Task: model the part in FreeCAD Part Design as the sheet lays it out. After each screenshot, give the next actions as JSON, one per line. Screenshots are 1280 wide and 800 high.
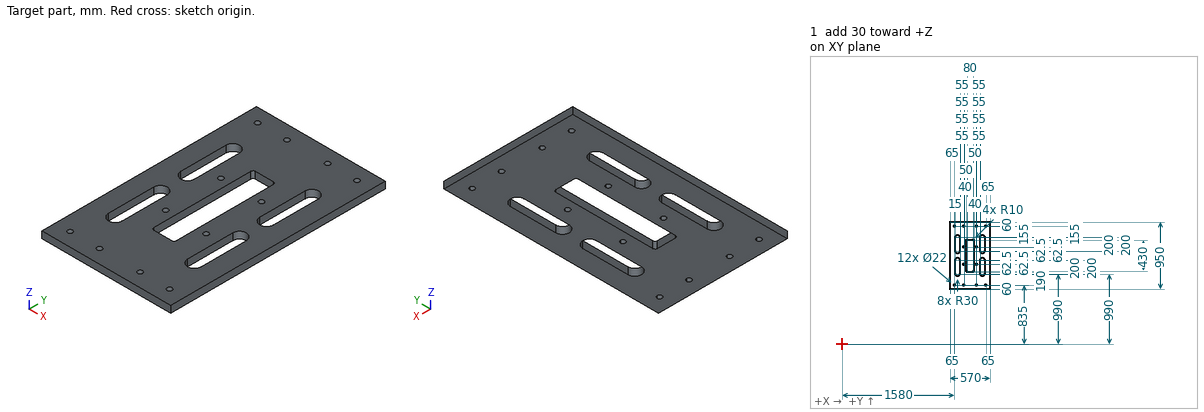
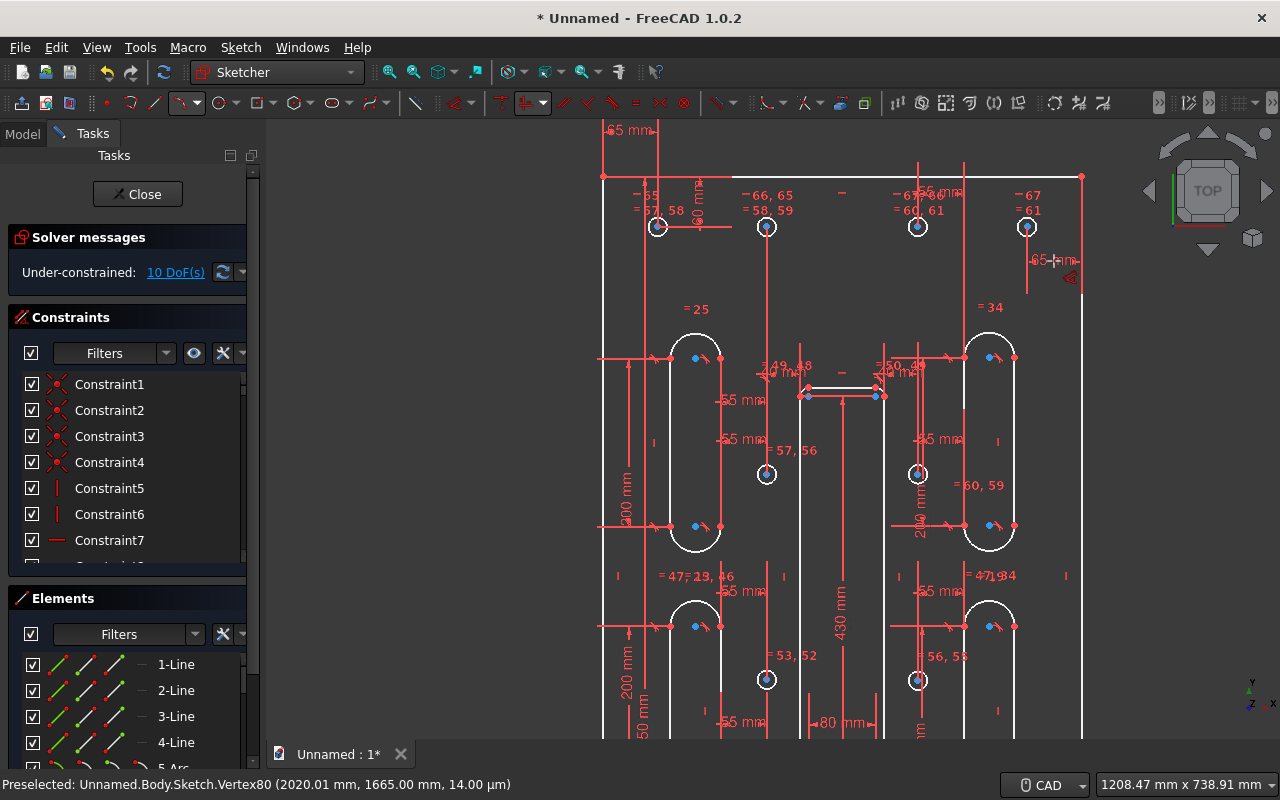
{"action": "scroll", "coordinate": [919, 226], "scroll_direction": "down", "scroll_amount": 6}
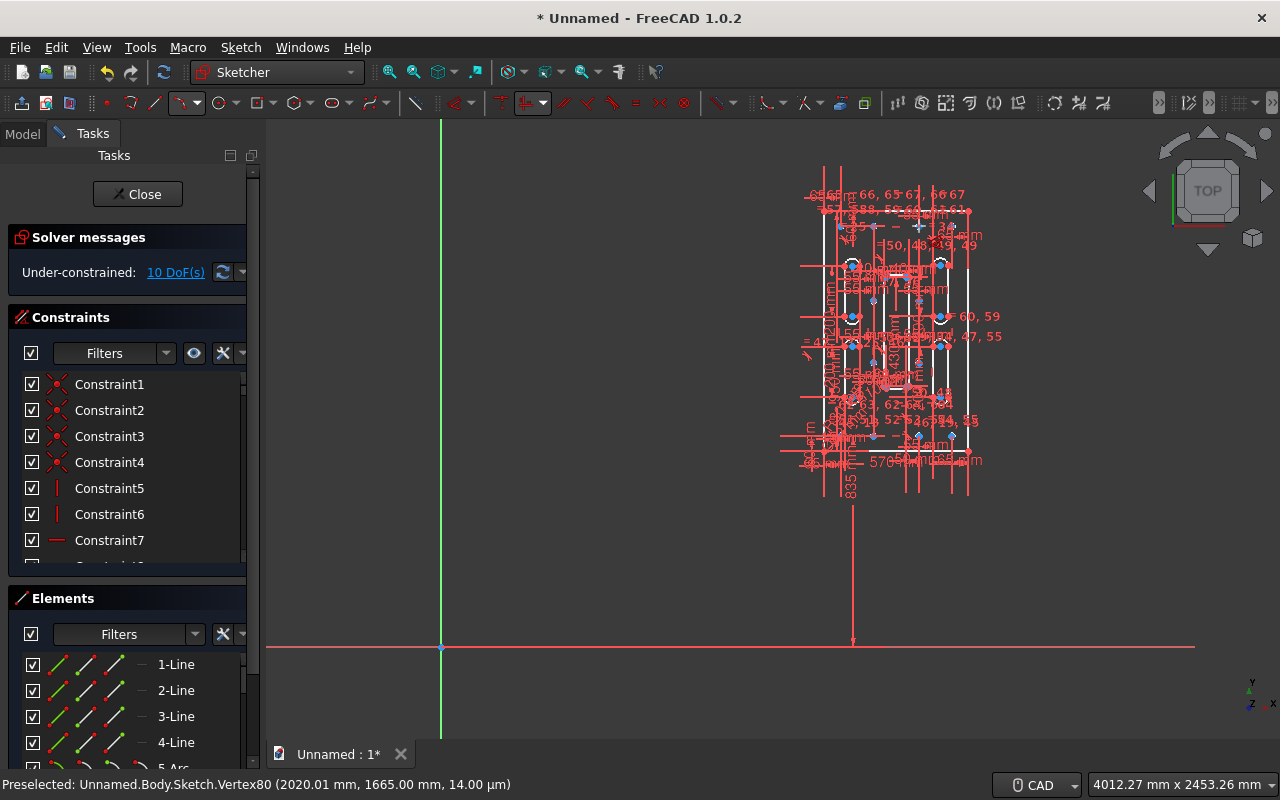
{"action": "scroll", "coordinate": [845, 397], "scroll_direction": "up", "scroll_amount": 3}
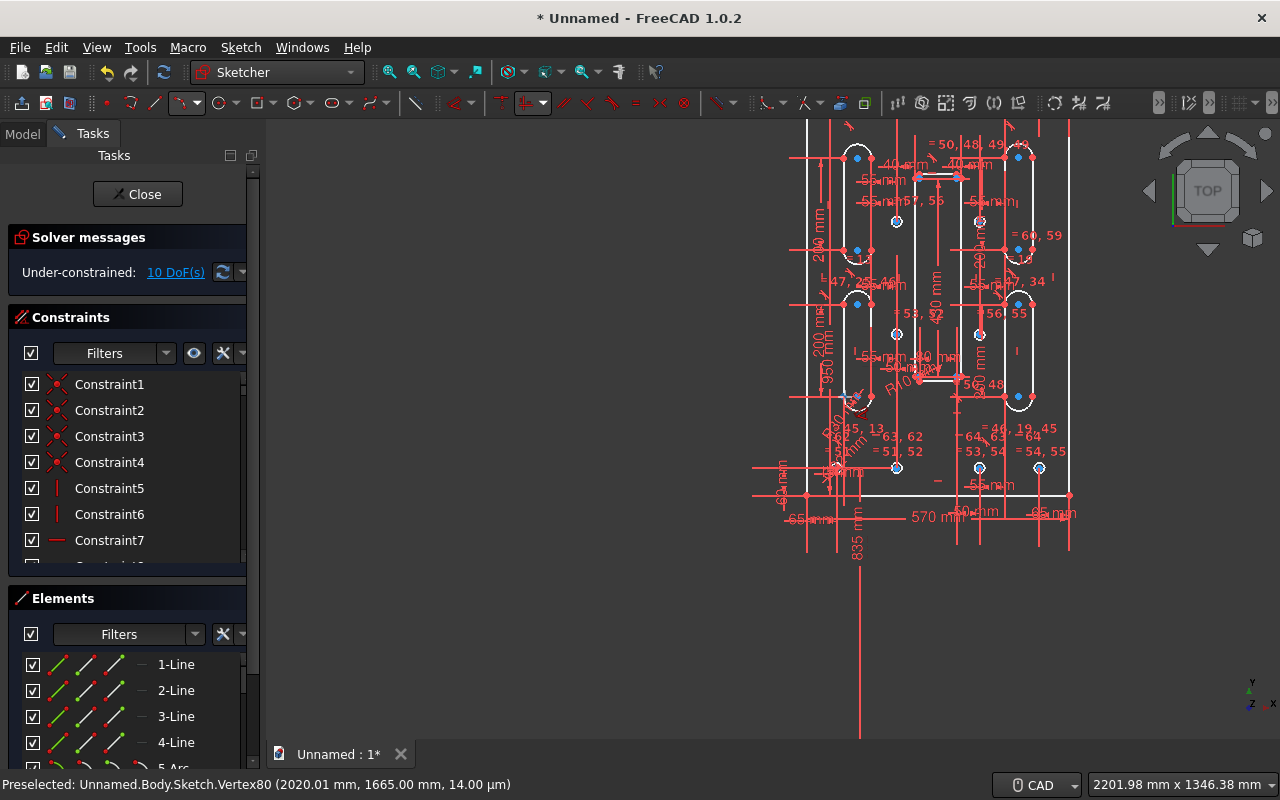
{"action": "left_click", "coordinate": [844, 397]}
{"action": "left_click", "coordinate": [878, 554]}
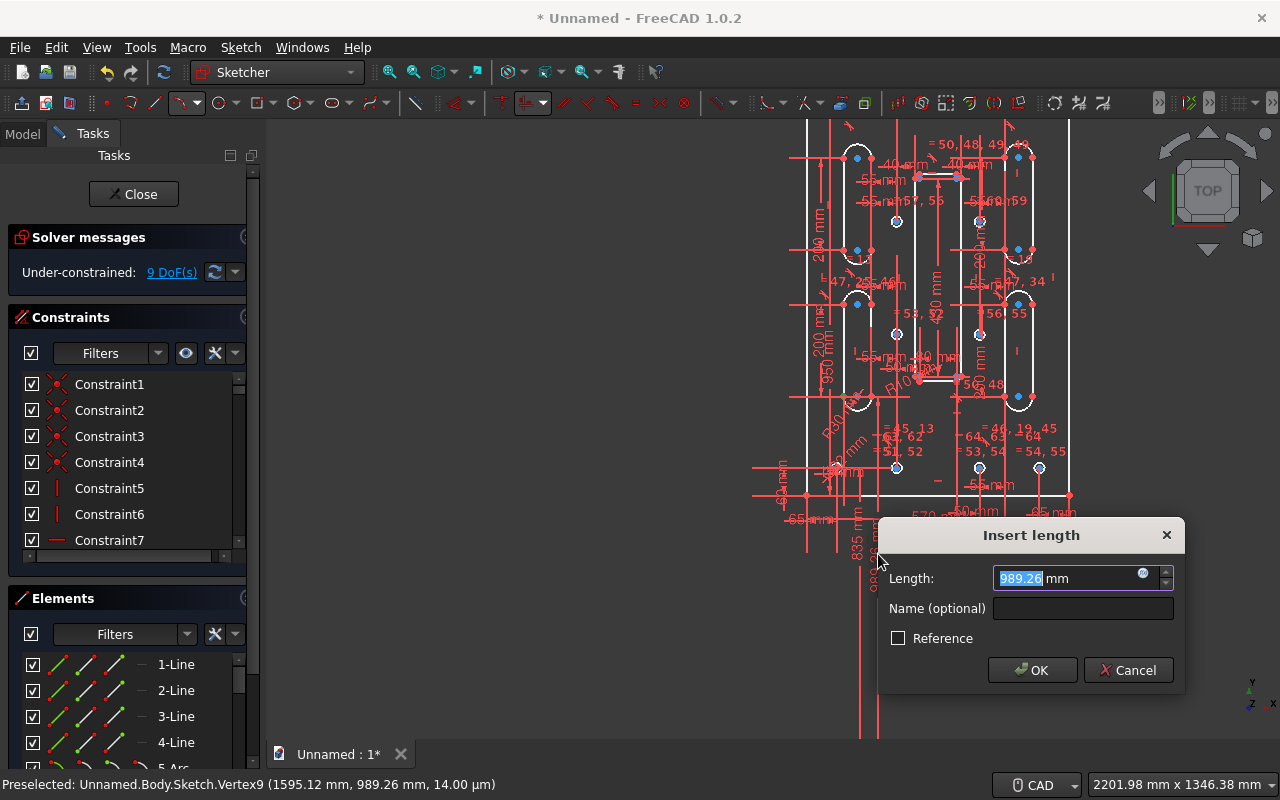
{"action": "type", "text": "990"}
{"action": "key", "text": "Return"}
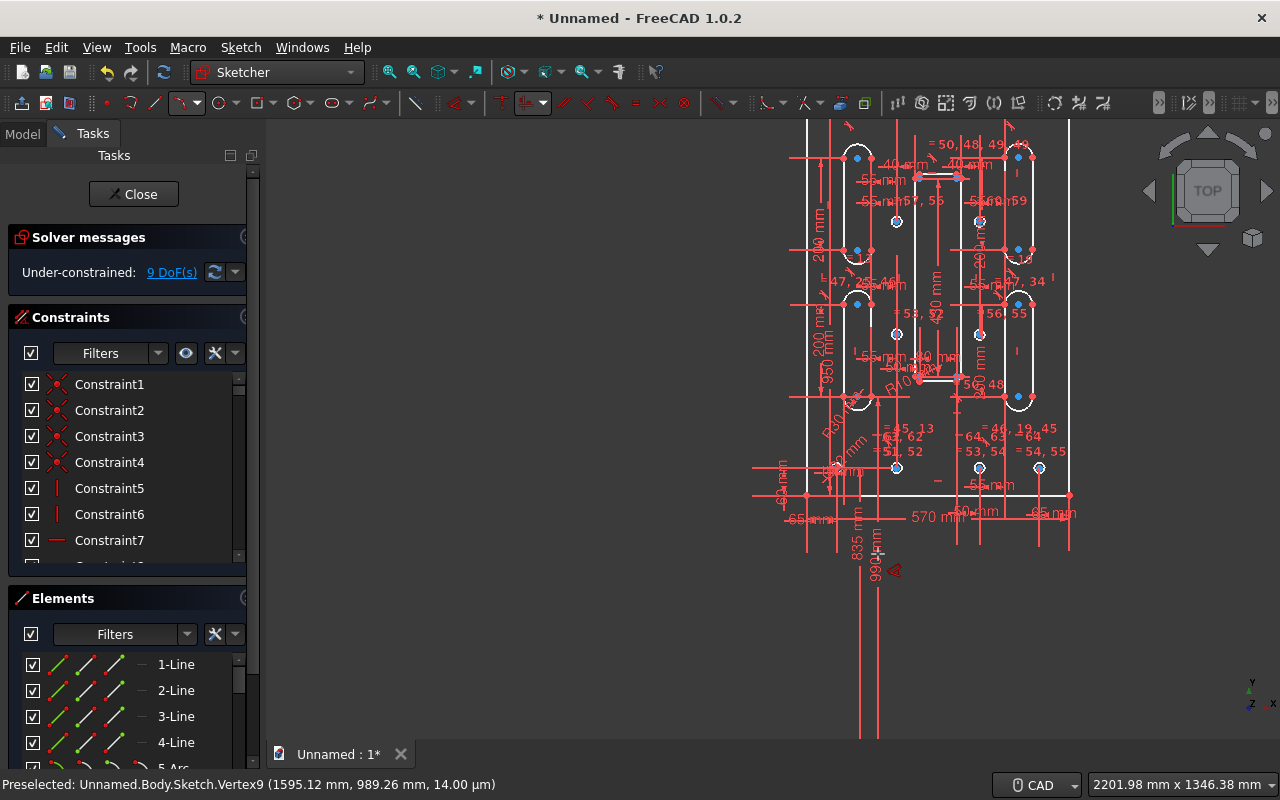
{"action": "left_click", "coordinate": [1005, 397]}
{"action": "left_click", "coordinate": [1039, 554]}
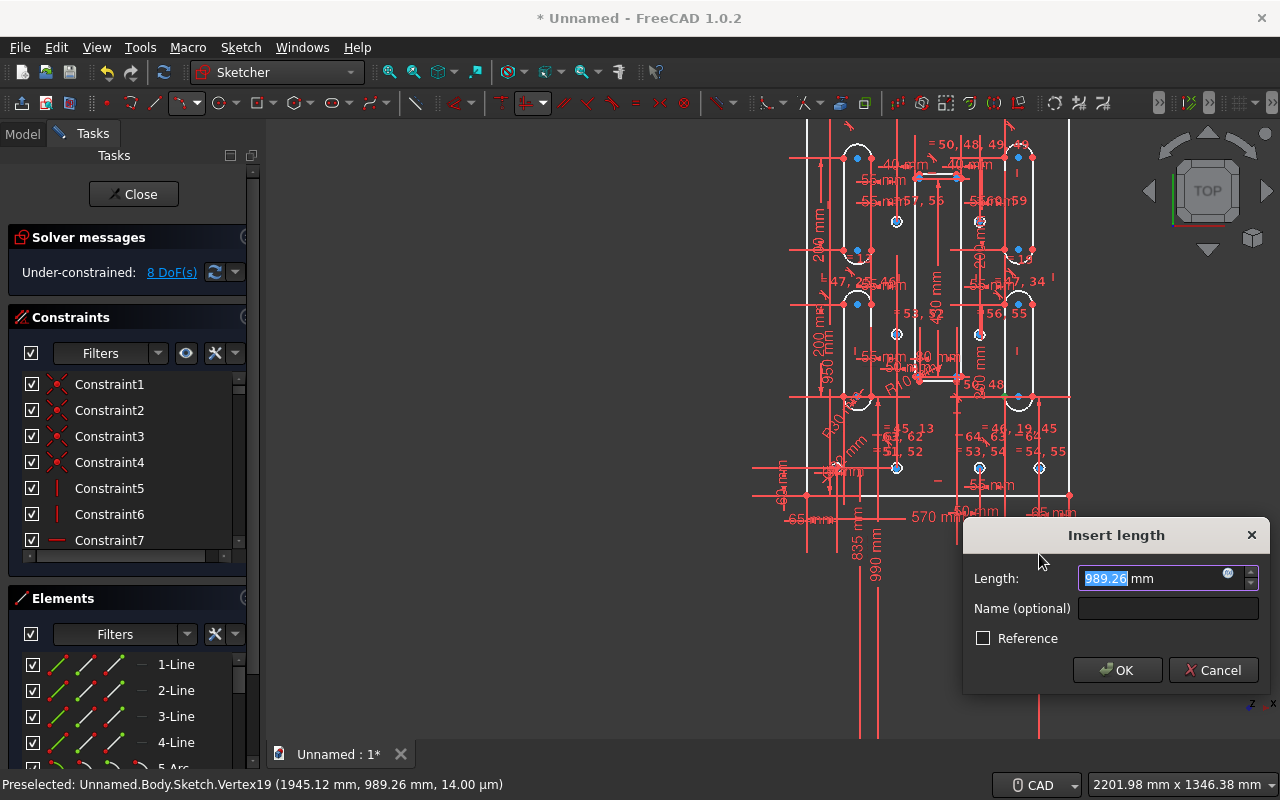
{"action": "type", "text": "990"}
{"action": "key", "text": "Return"}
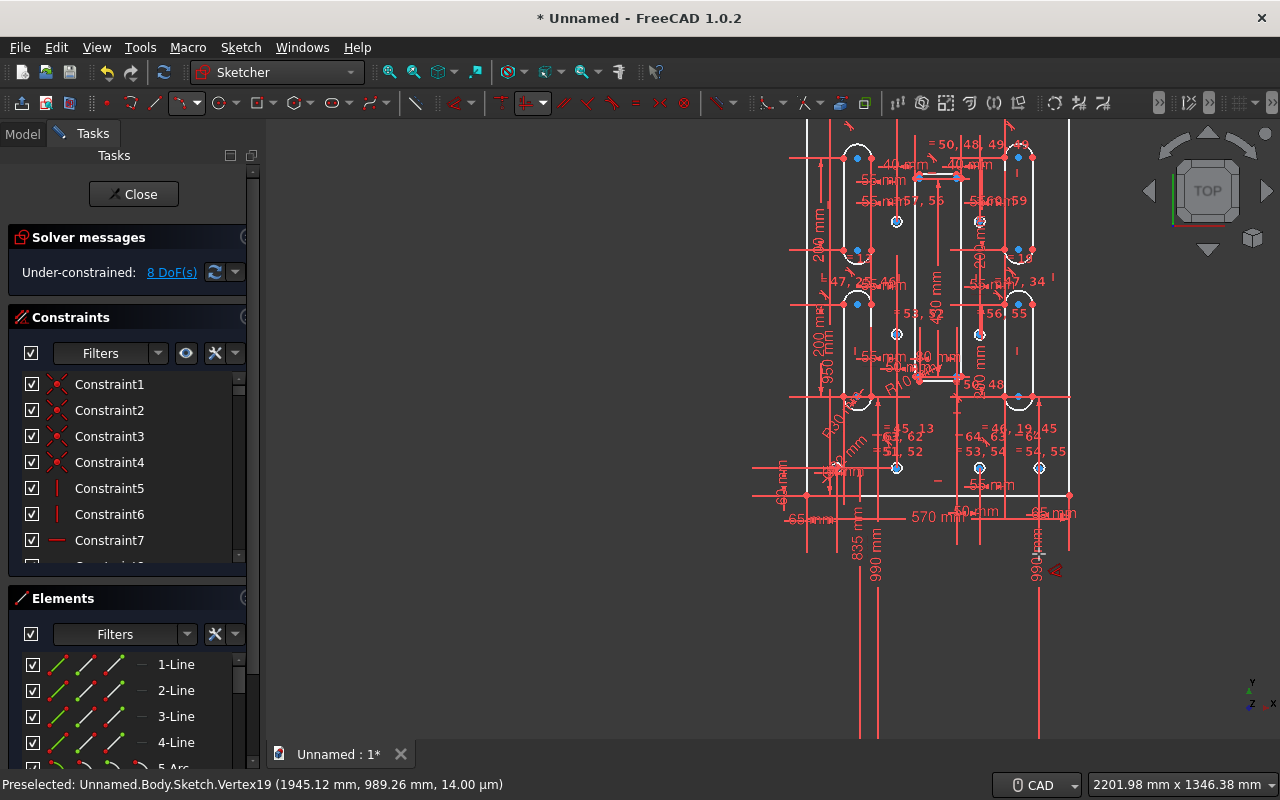
{"action": "left_click", "coordinate": [837, 468]}
{"action": "left_click", "coordinate": [565, 434]}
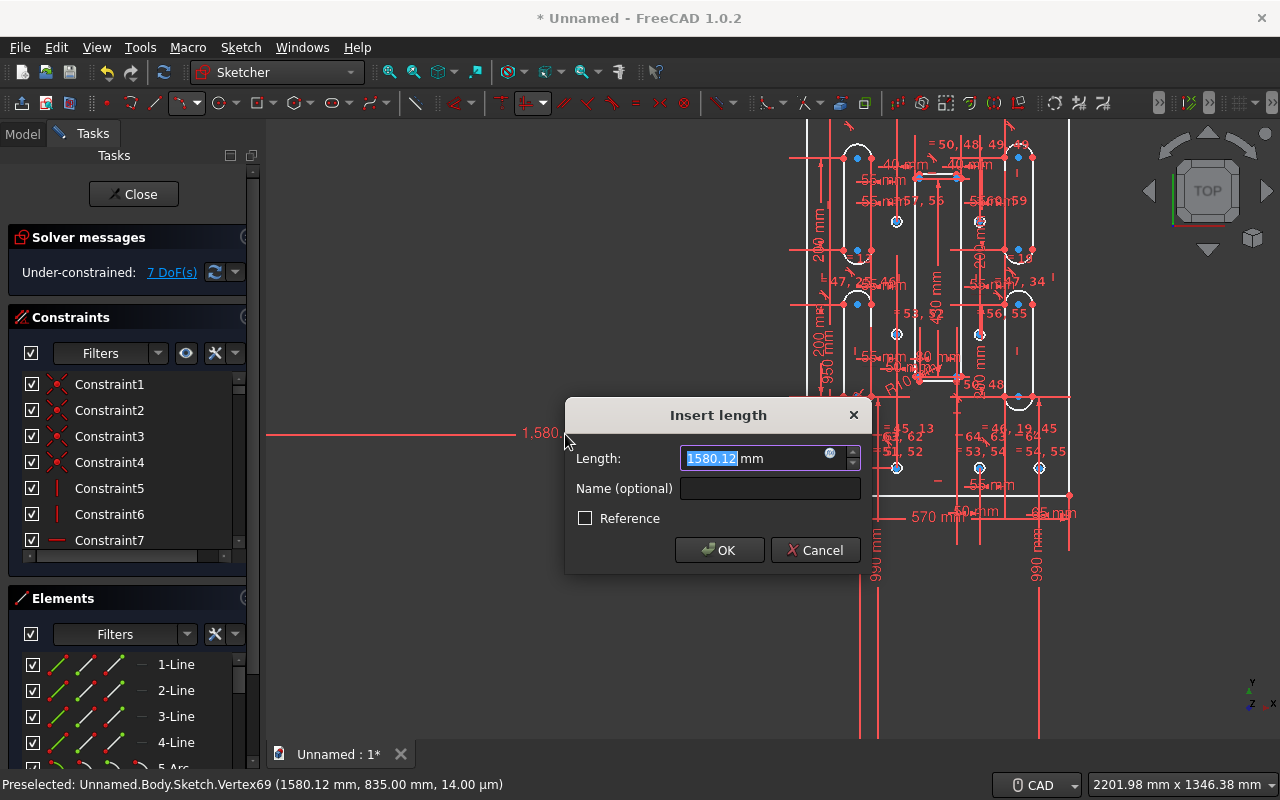
{"action": "type", "text": "1580"}
{"action": "key", "text": "Return"}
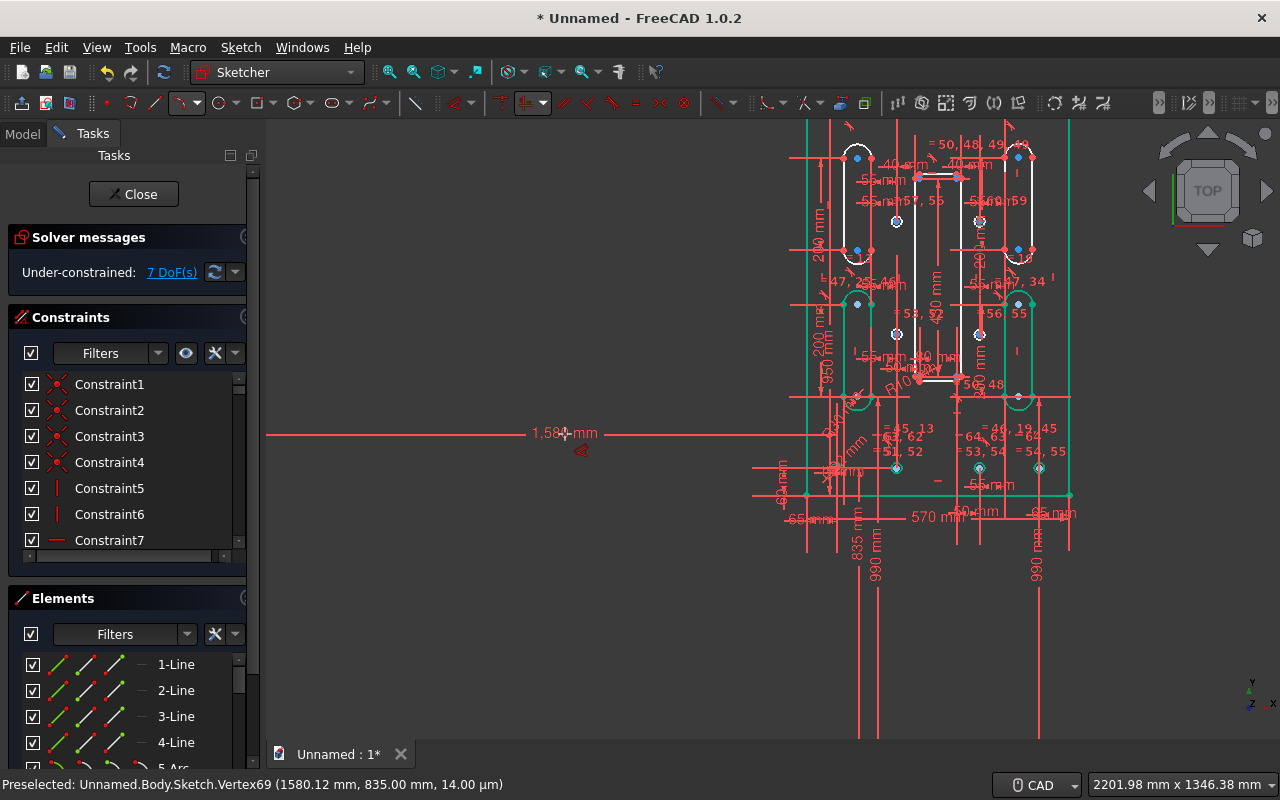
{"action": "scroll", "coordinate": [920, 381], "scroll_direction": "up", "scroll_amount": 5}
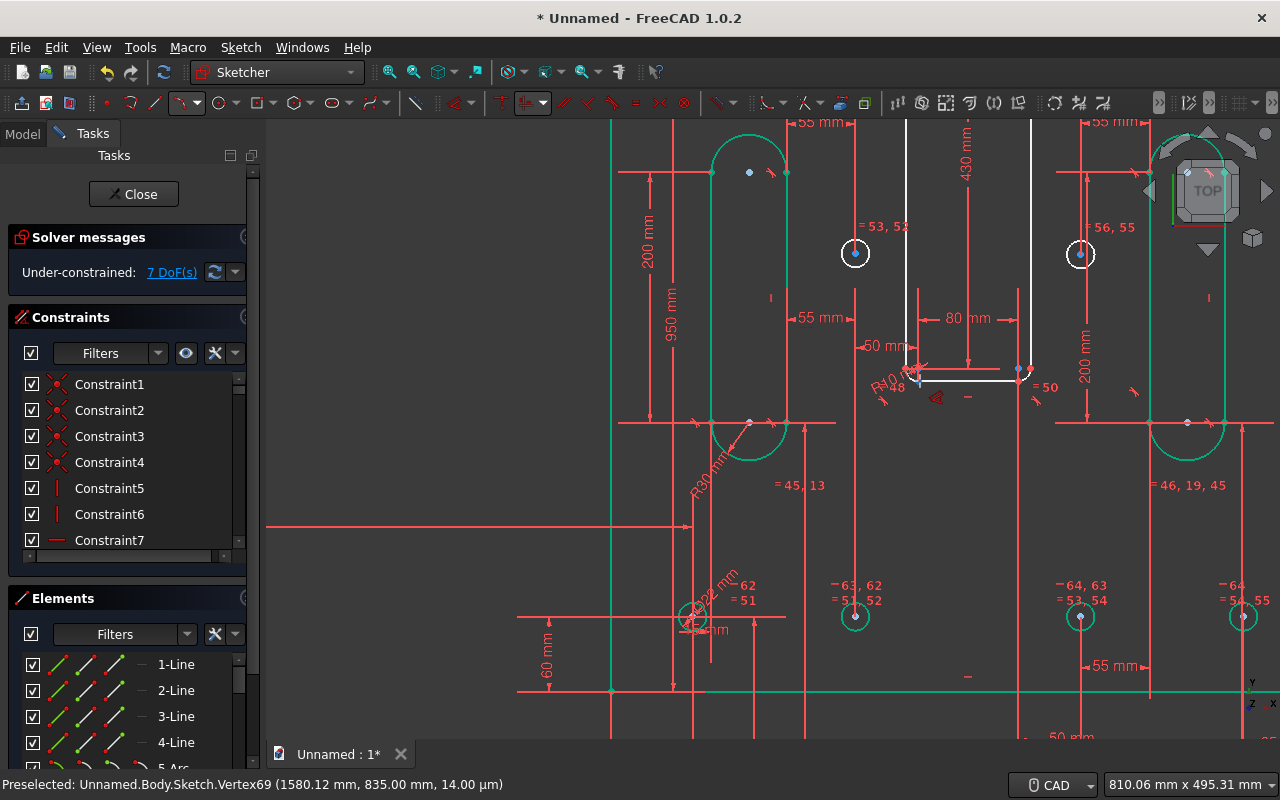
{"action": "left_click", "coordinate": [918, 381]}